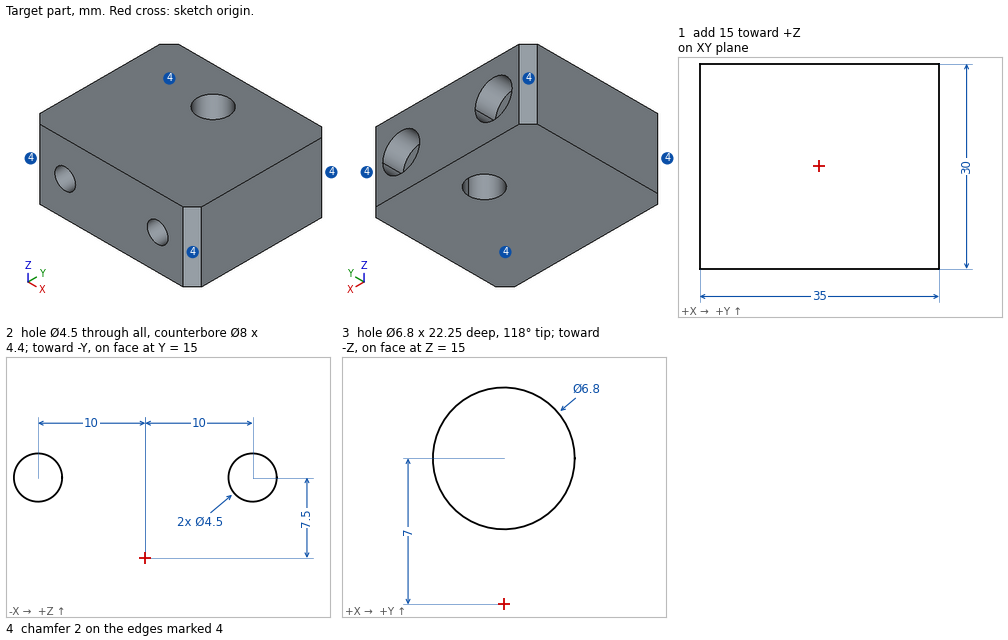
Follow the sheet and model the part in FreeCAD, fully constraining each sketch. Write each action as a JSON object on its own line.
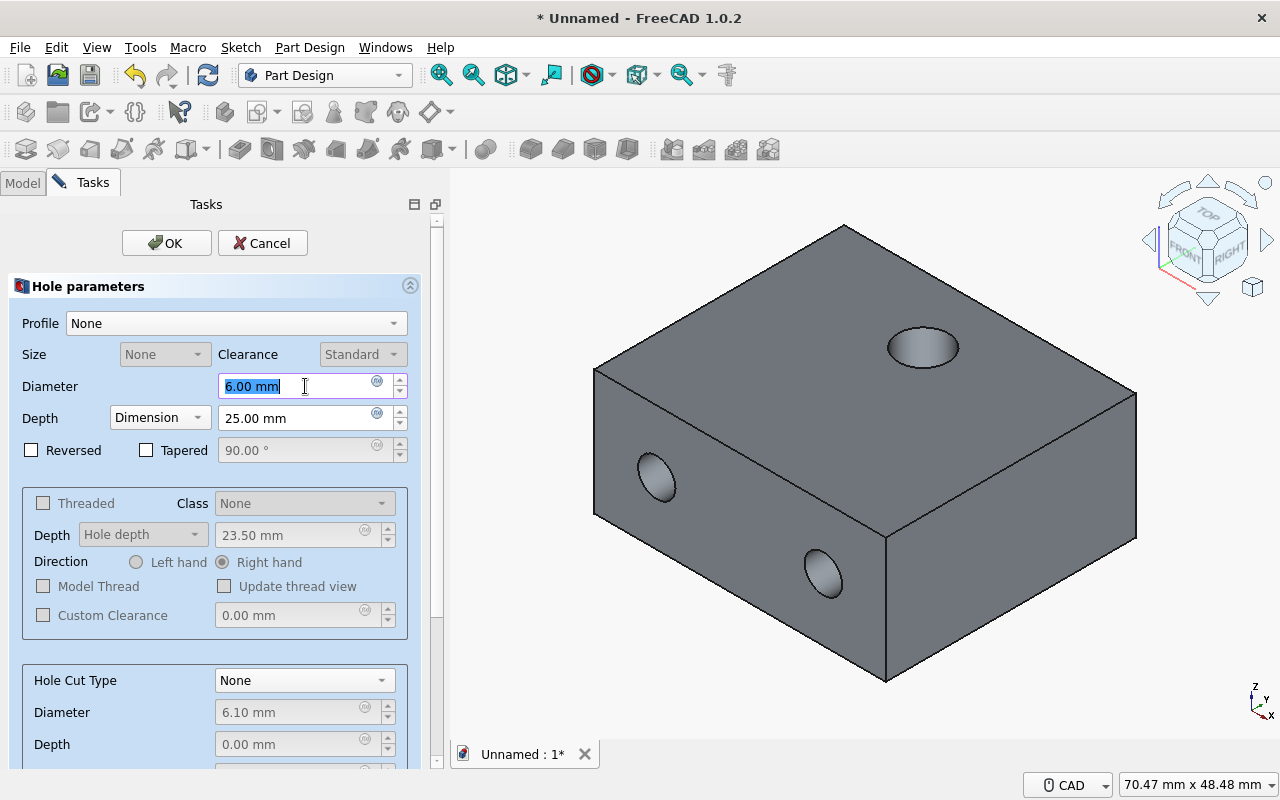
{"action": "type", "text": "6.8"}
{"action": "key", "text": "Tab"}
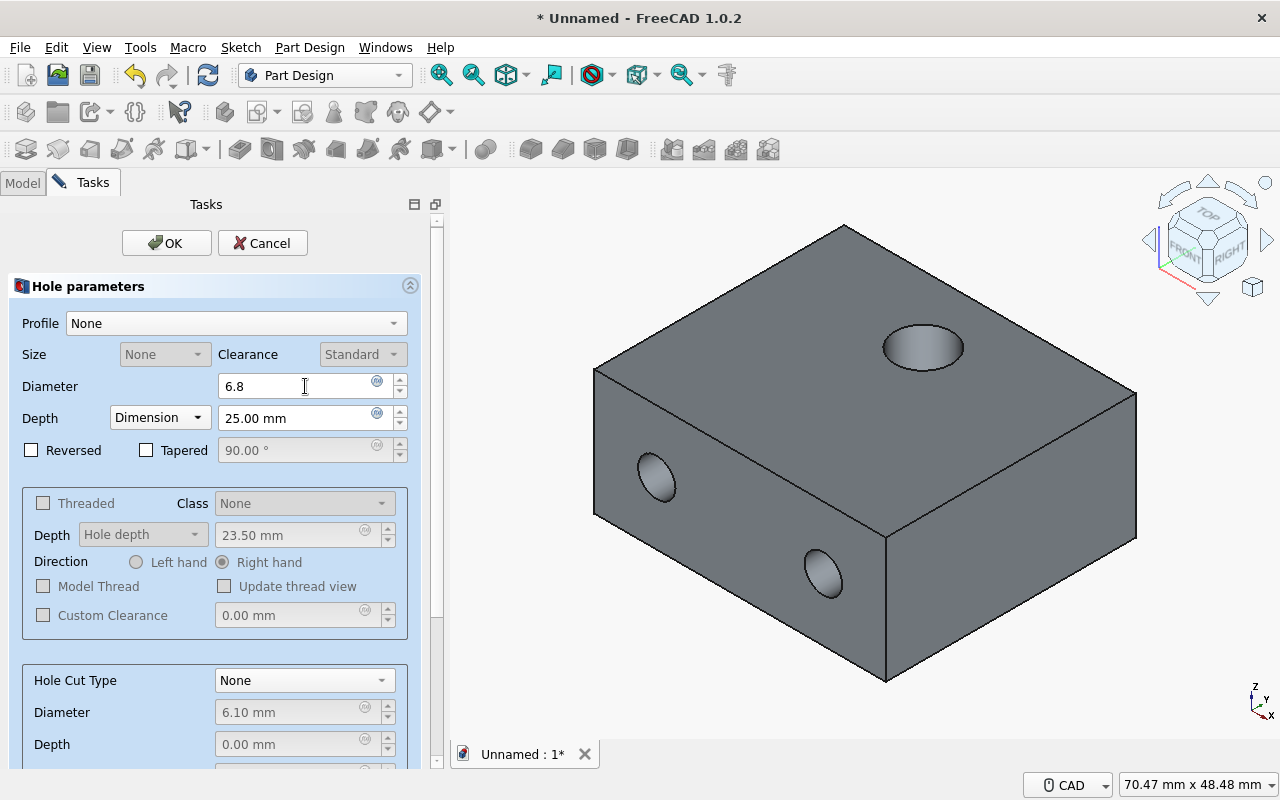
{"action": "triple_click", "coordinate": [305, 418]}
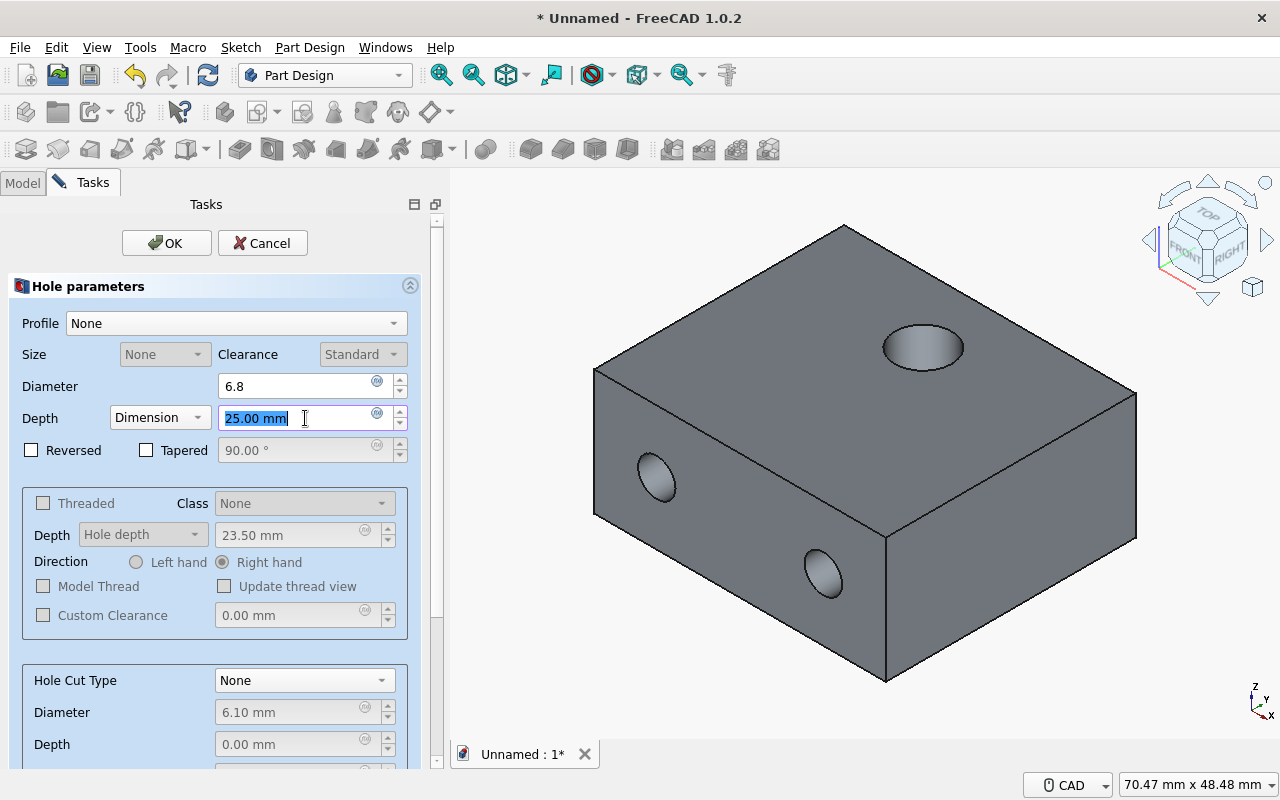
{"action": "type", "text": "22.25"}
{"action": "key", "text": "Tab"}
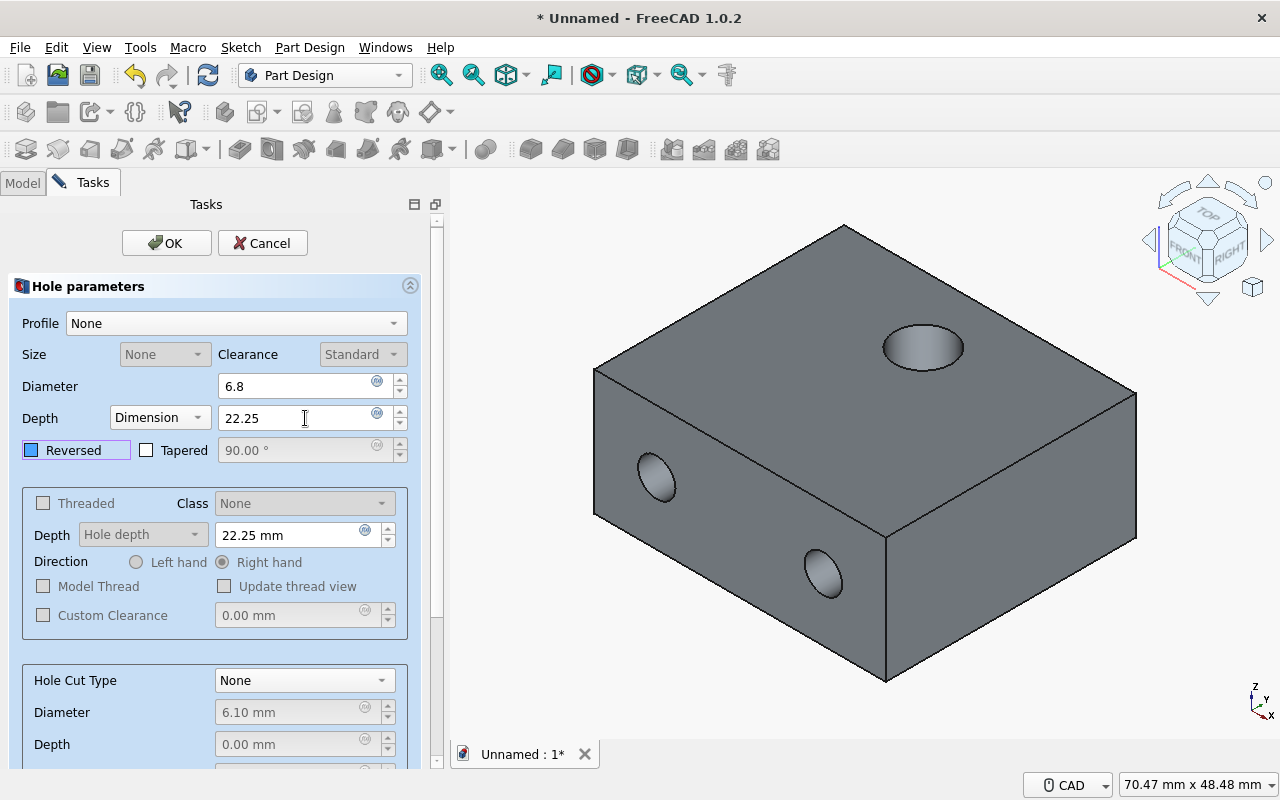
{"action": "left_click", "coordinate": [167, 243]}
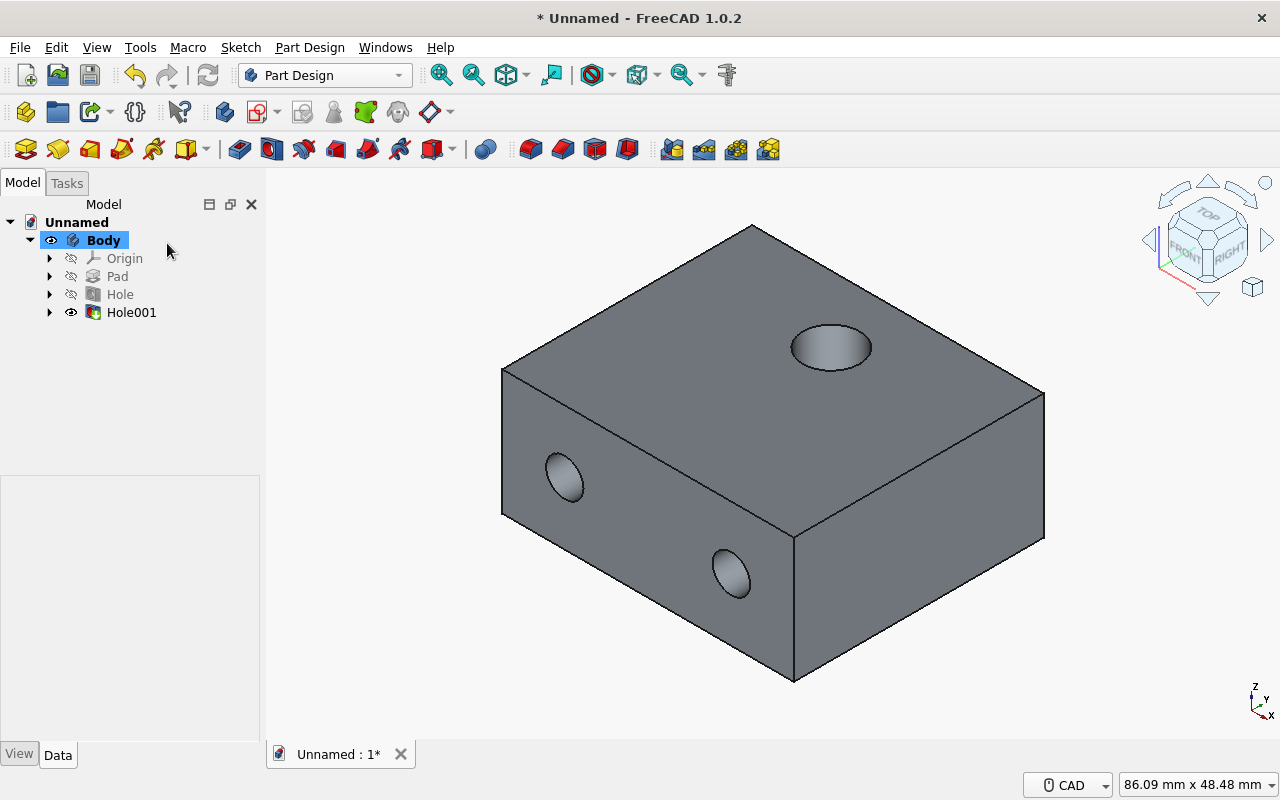
{"action": "left_click", "coordinate": [794, 609]}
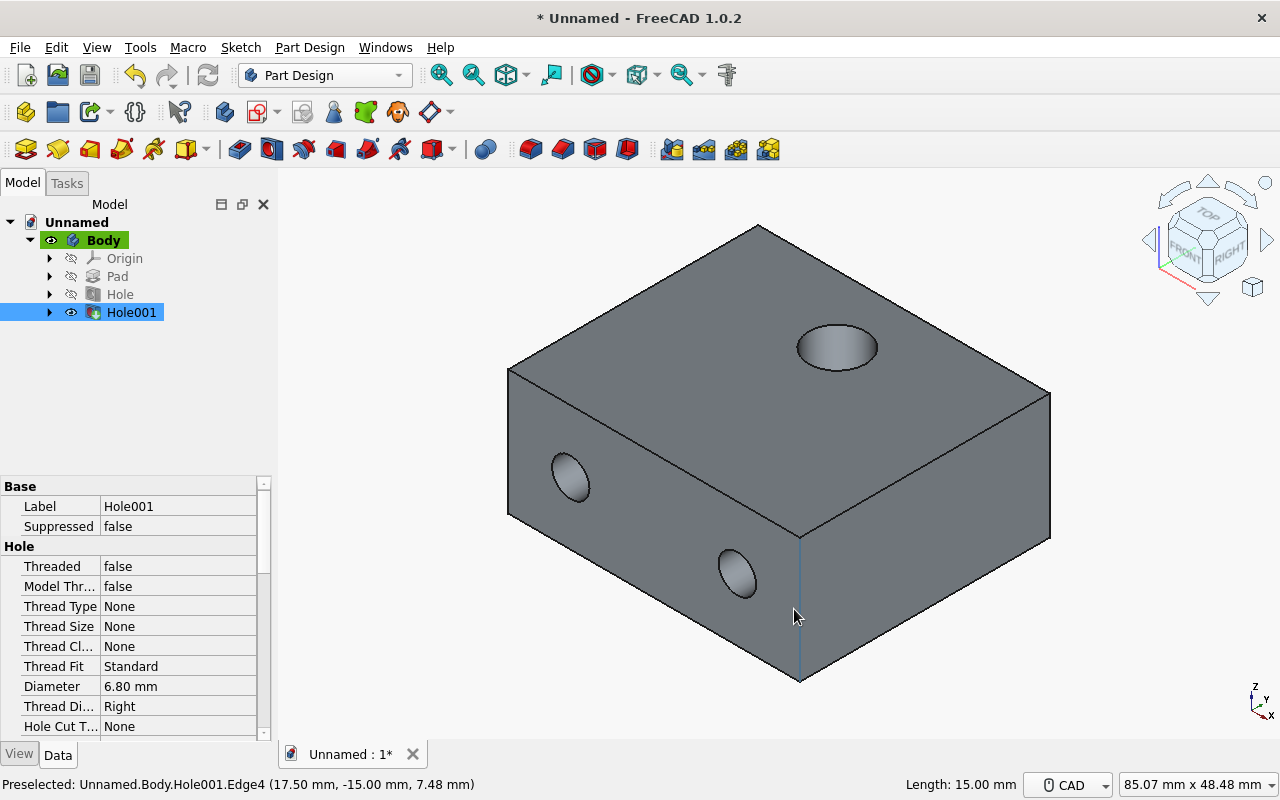
{"action": "key", "text": "2"}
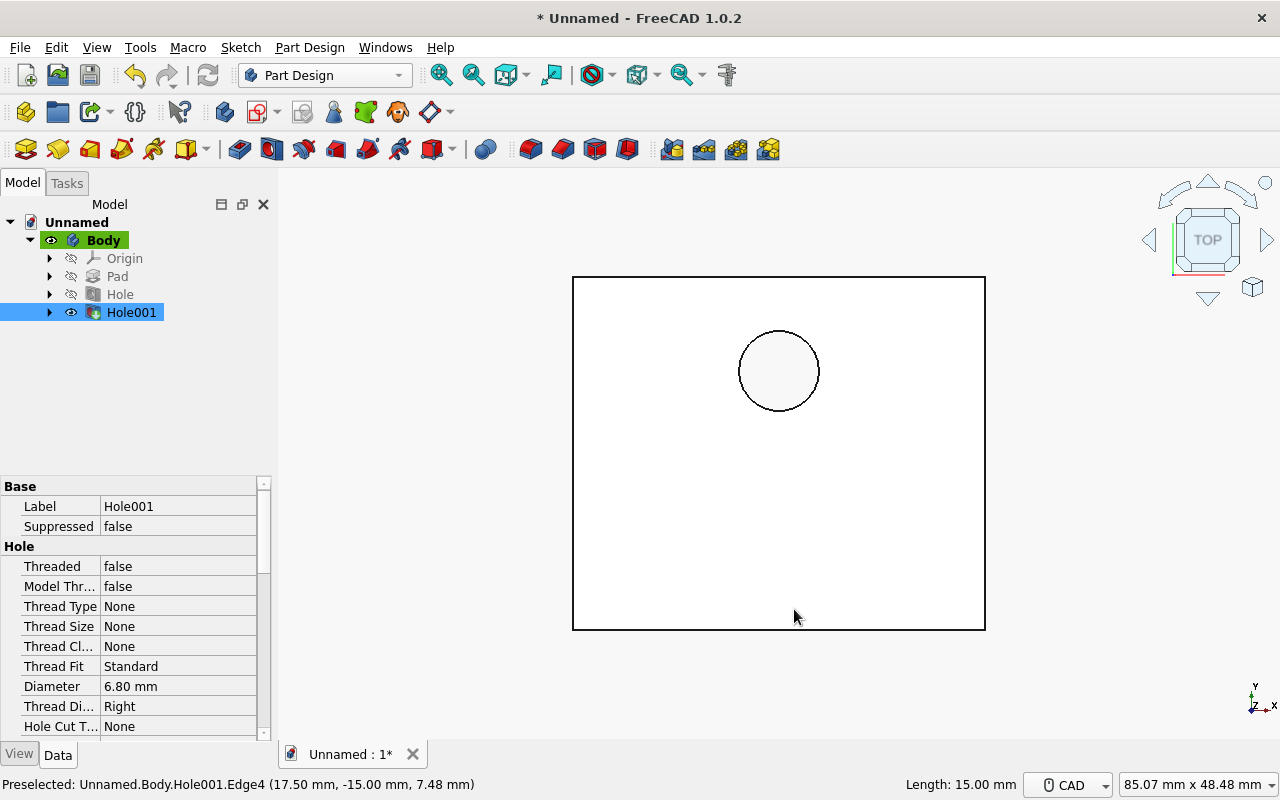
{"action": "key", "text": "0"}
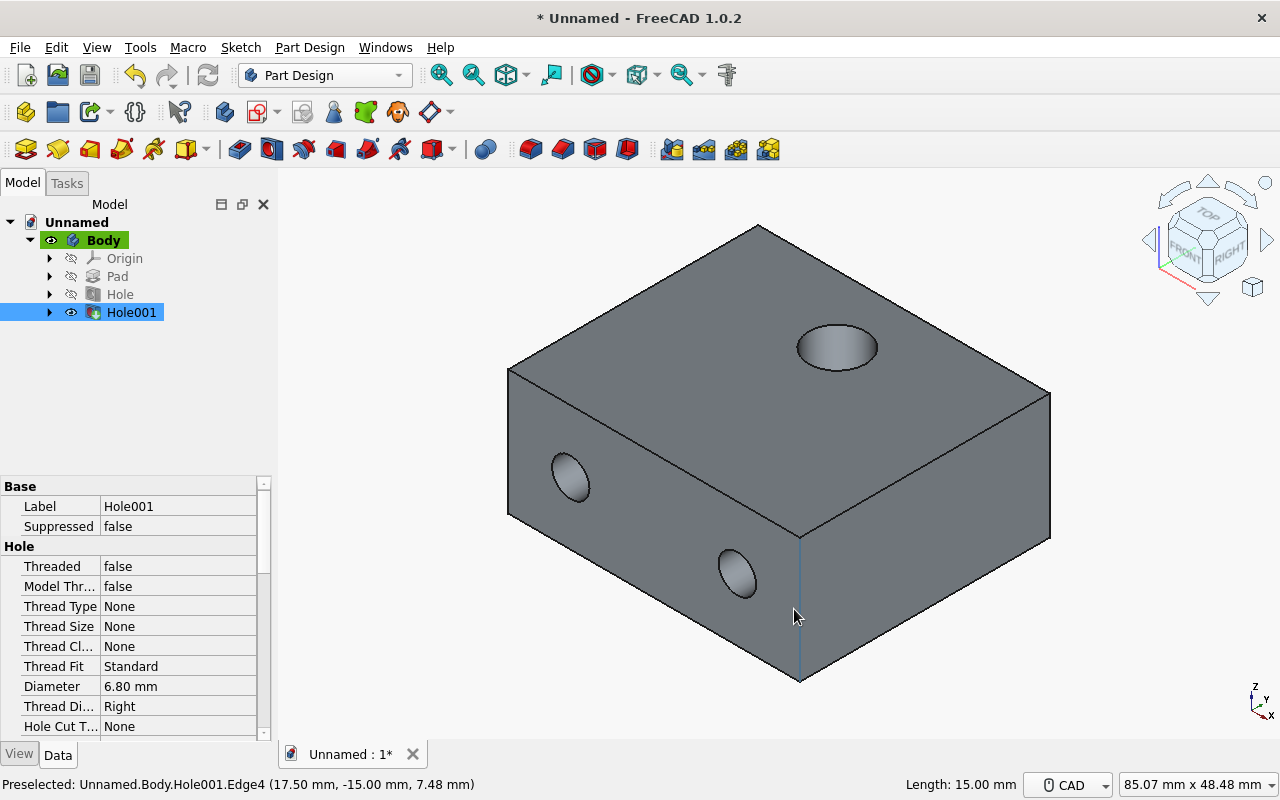
{"action": "key", "text": "1"}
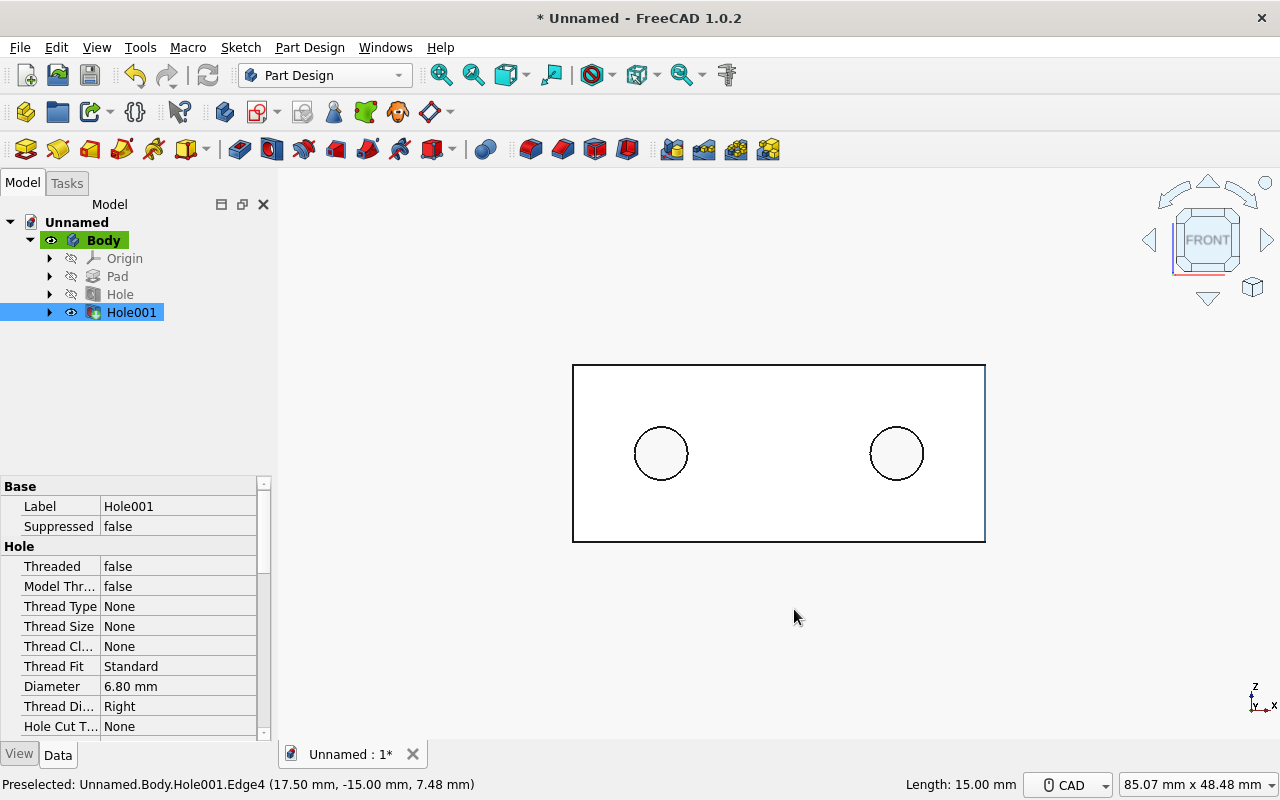
{"action": "key", "text": "v f"}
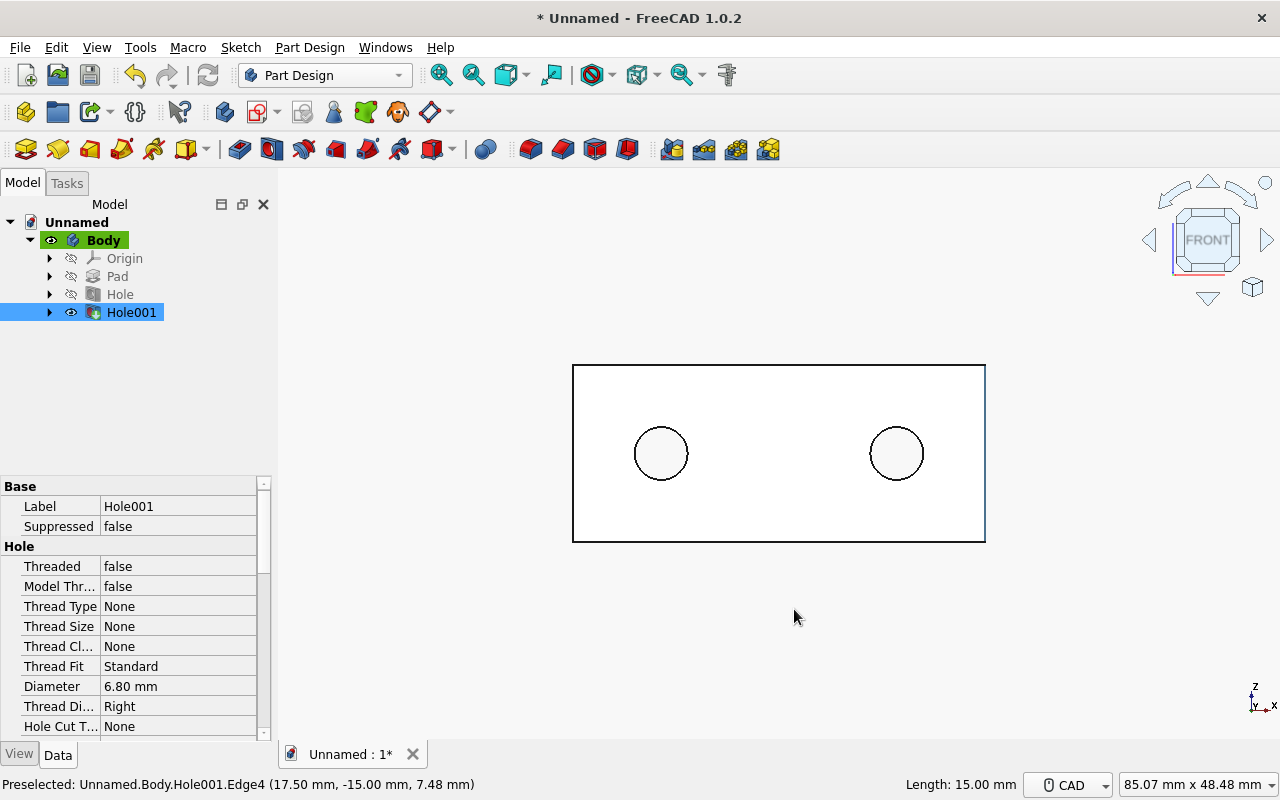
{"action": "left_click", "coordinate": [573, 453], "text": "ctrl"}